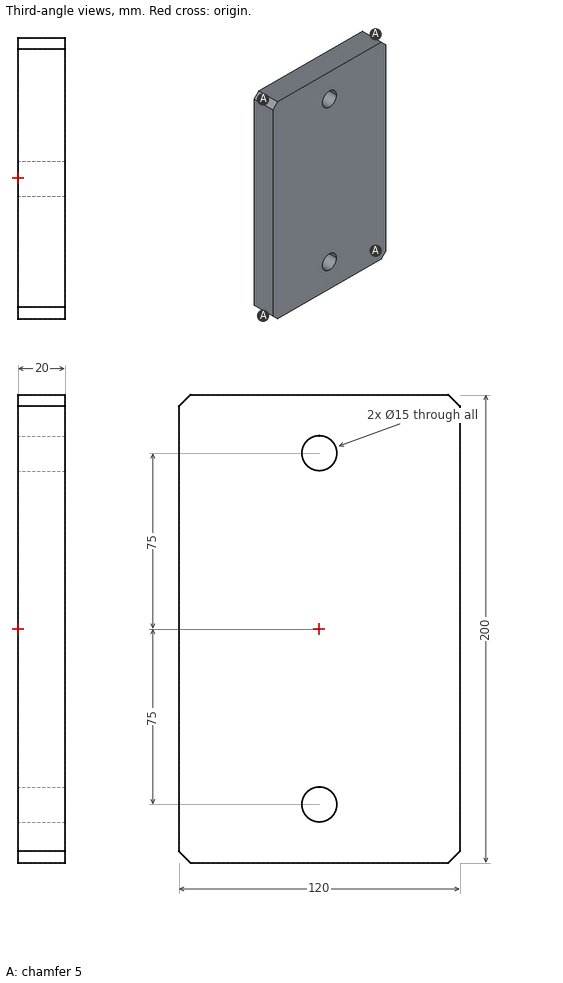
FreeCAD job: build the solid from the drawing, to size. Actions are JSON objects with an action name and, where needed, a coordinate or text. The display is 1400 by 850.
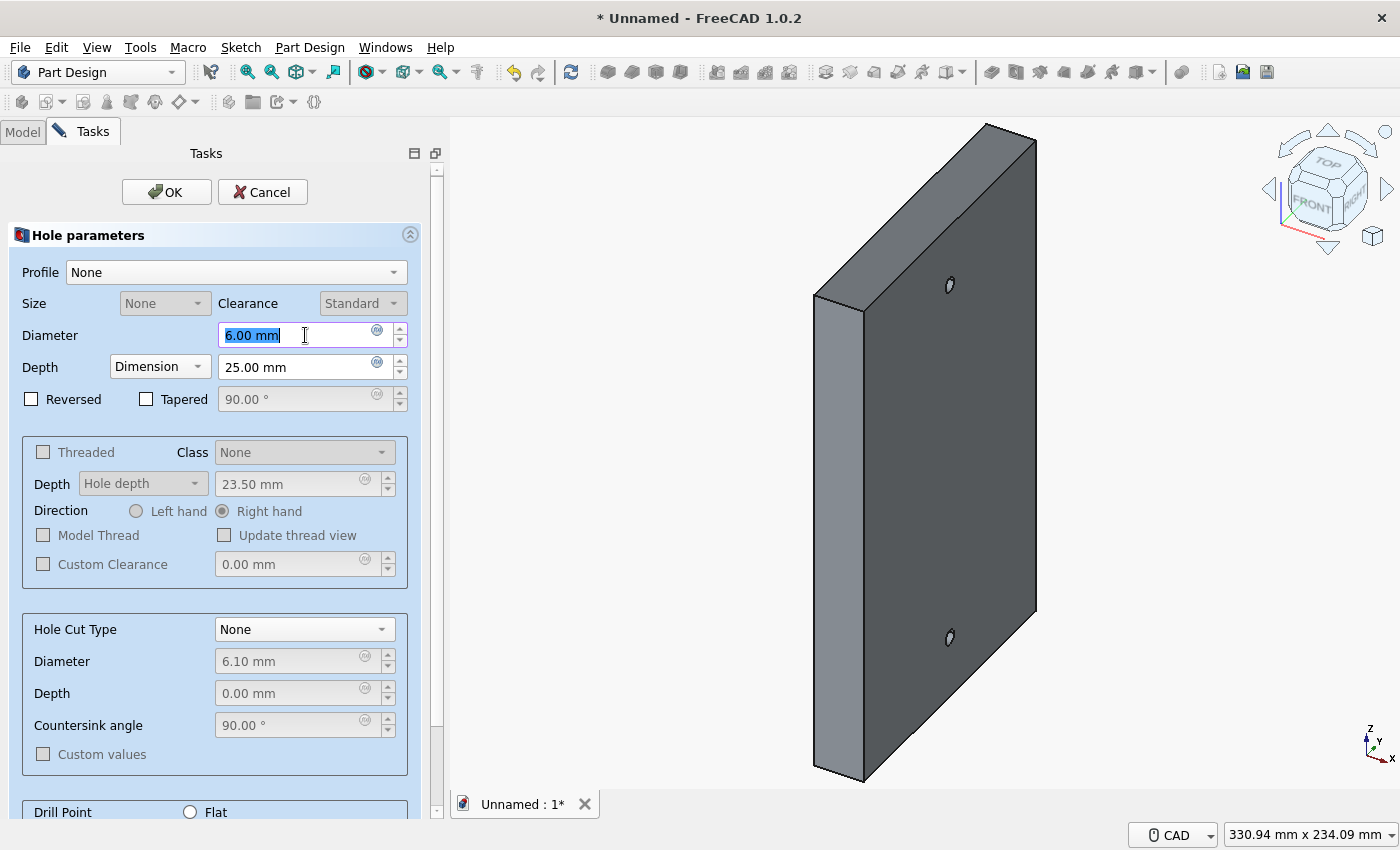
{"action": "type", "text": "15"}
{"action": "key", "text": "Tab"}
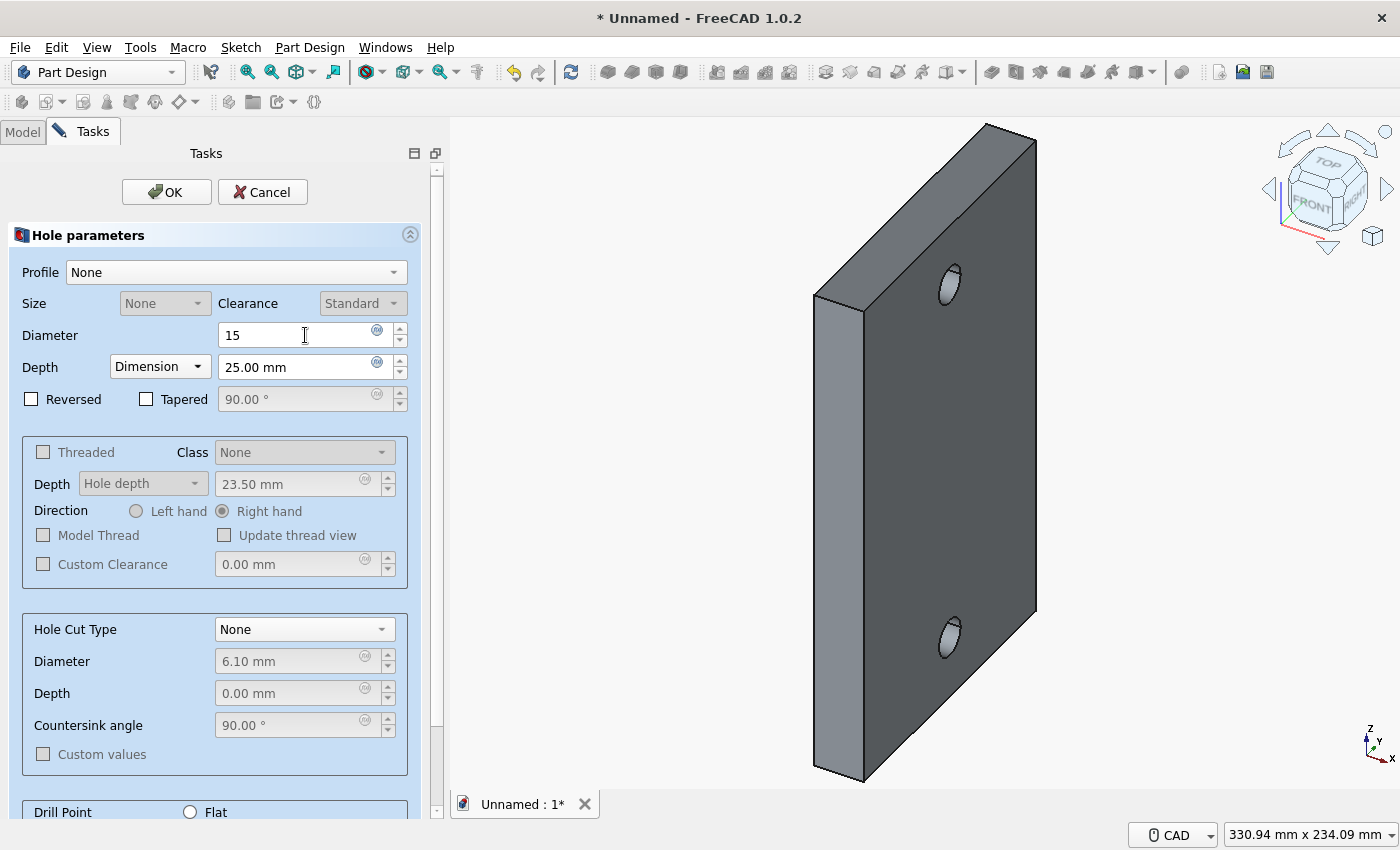
{"action": "left_click", "coordinate": [161, 366]}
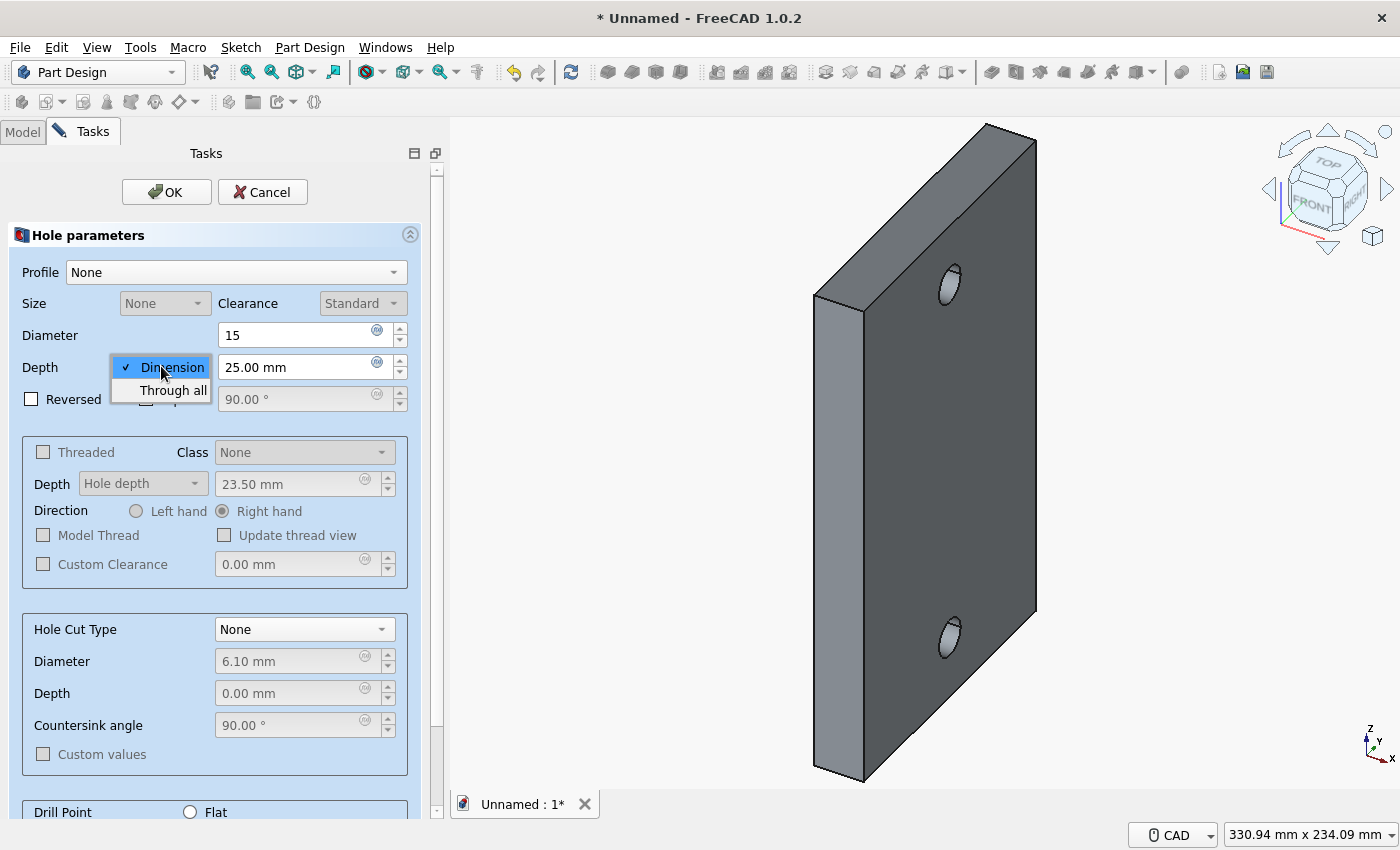
{"action": "left_click", "coordinate": [160, 390]}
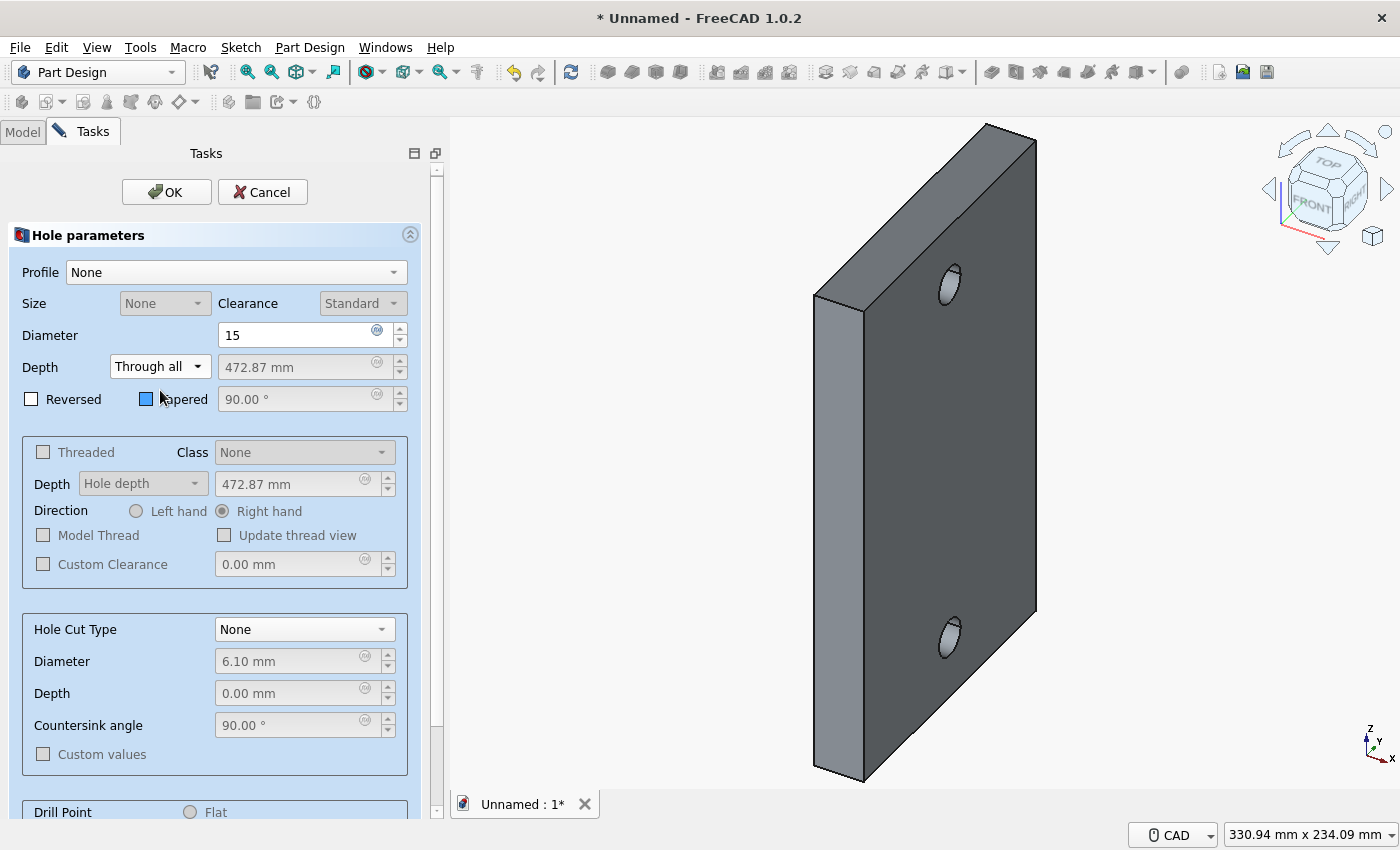
{"action": "left_click", "coordinate": [167, 192]}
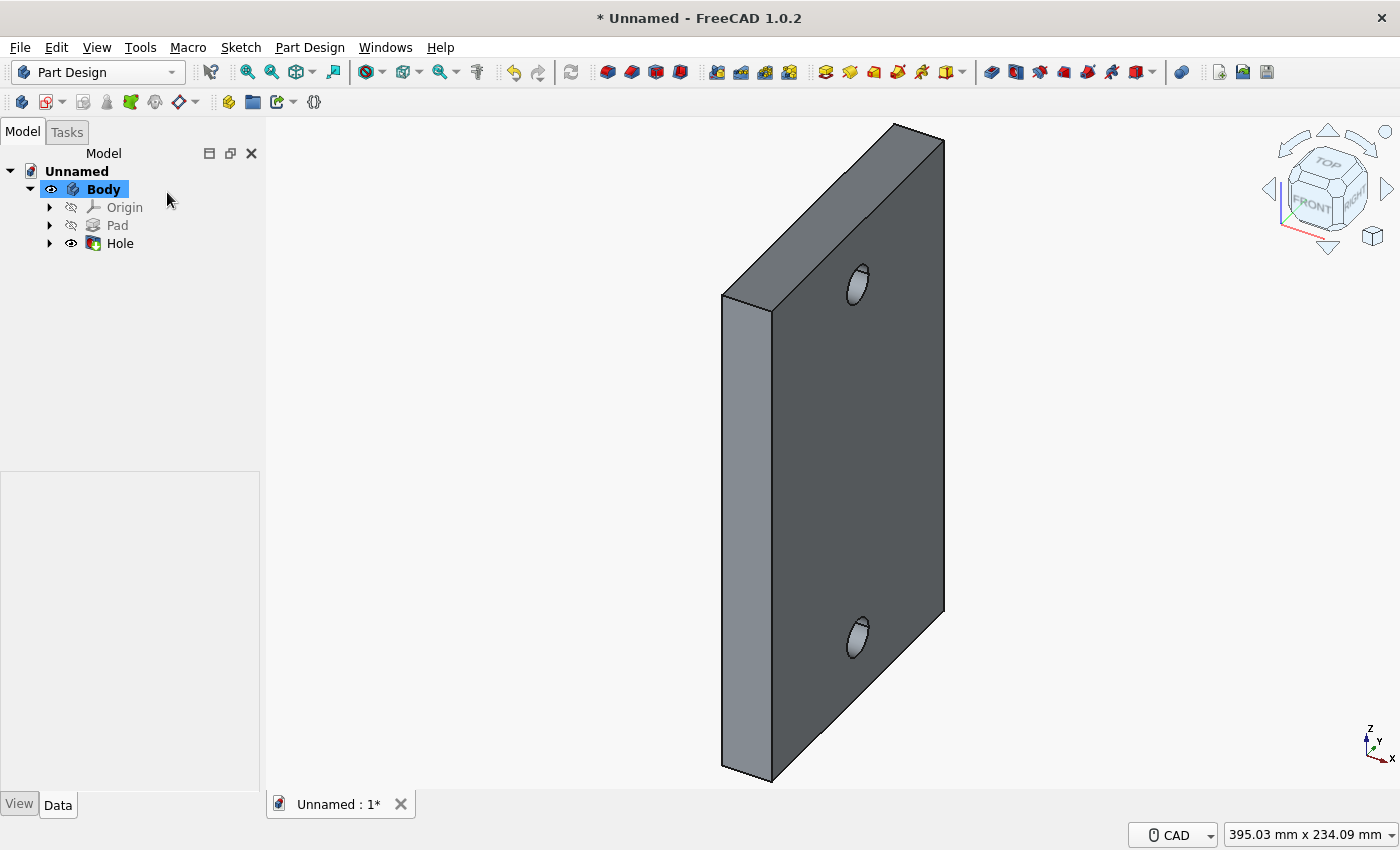
{"action": "left_click", "coordinate": [747, 302]}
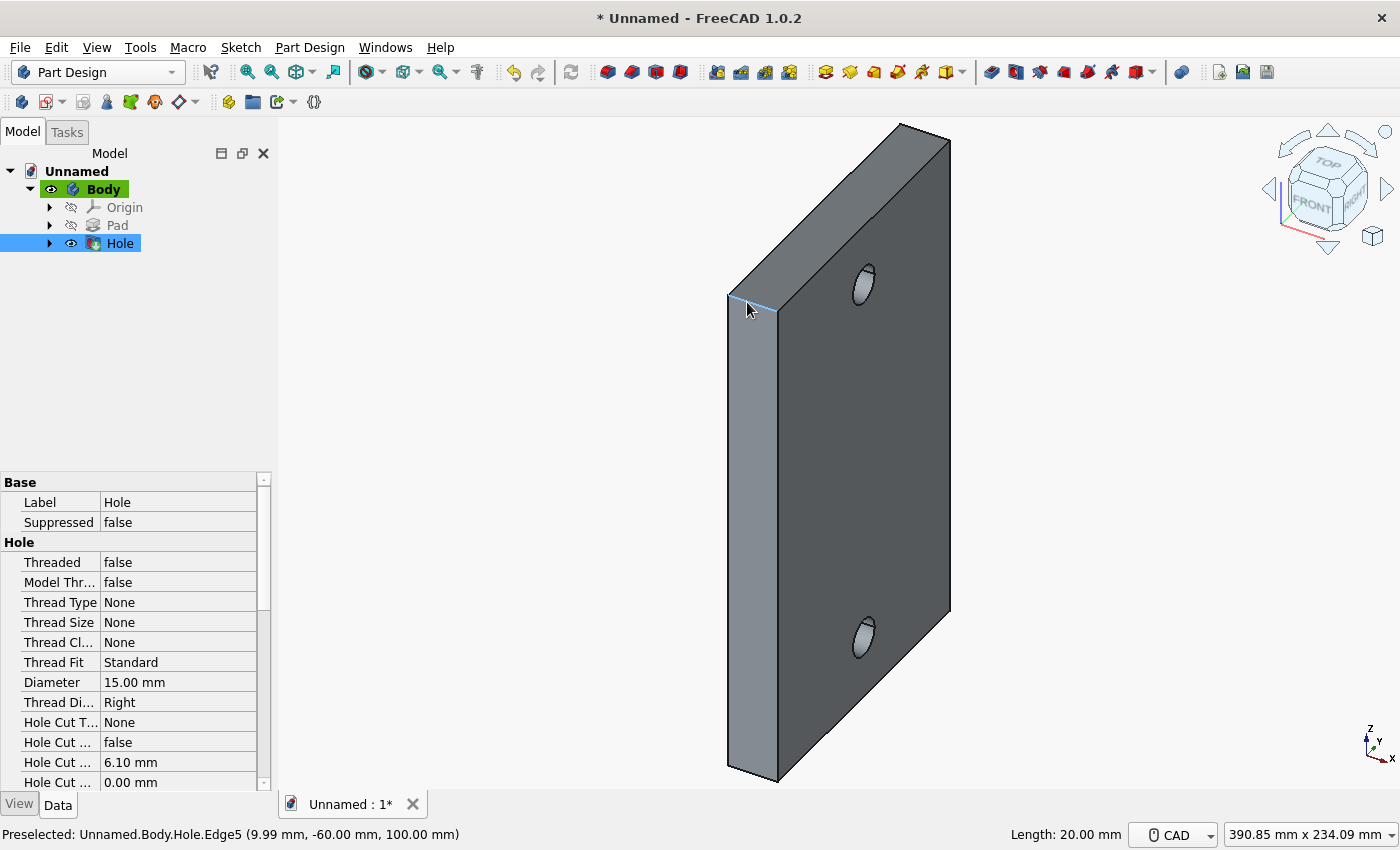
{"action": "key", "text": "0"}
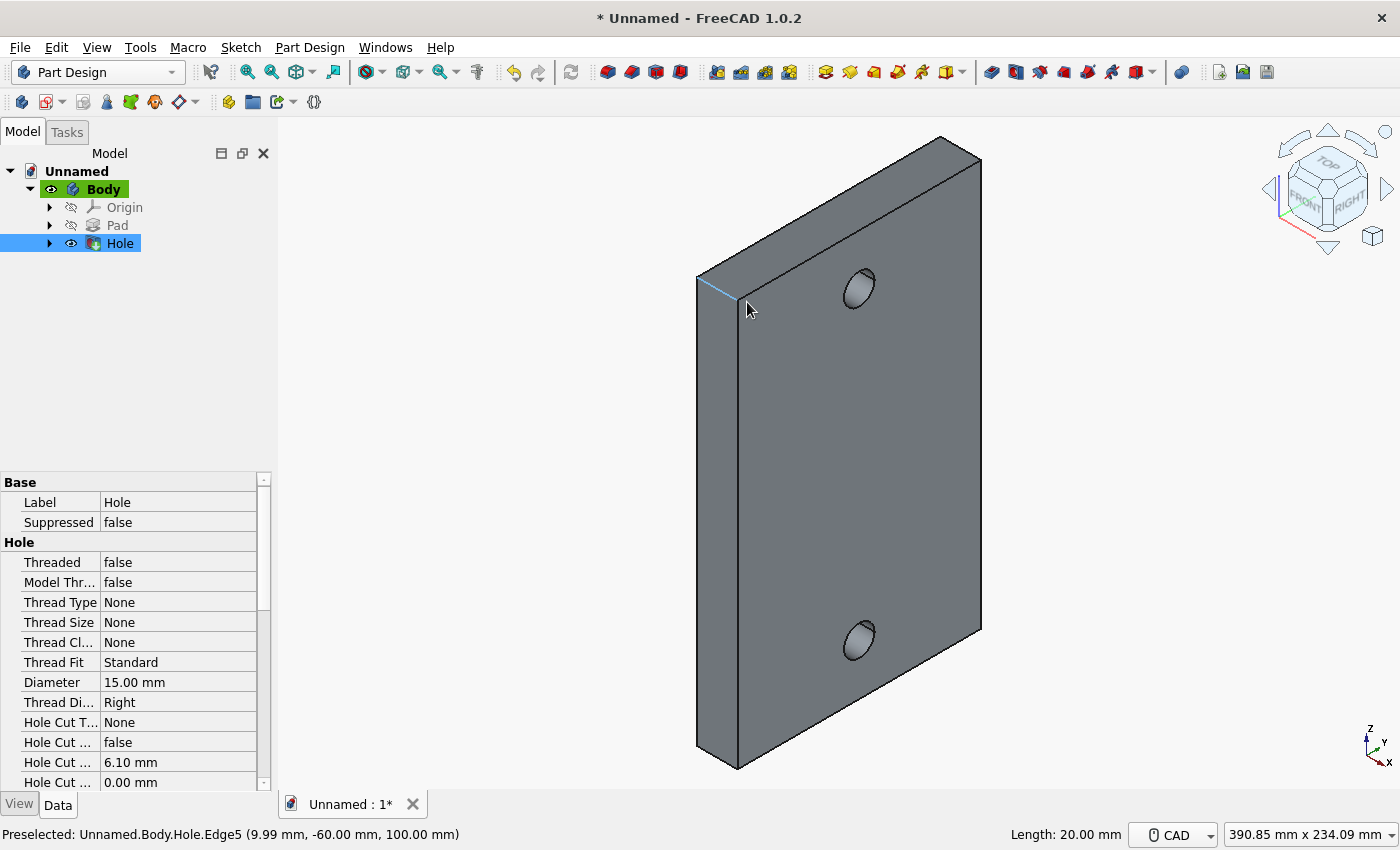
{"action": "key", "text": "2"}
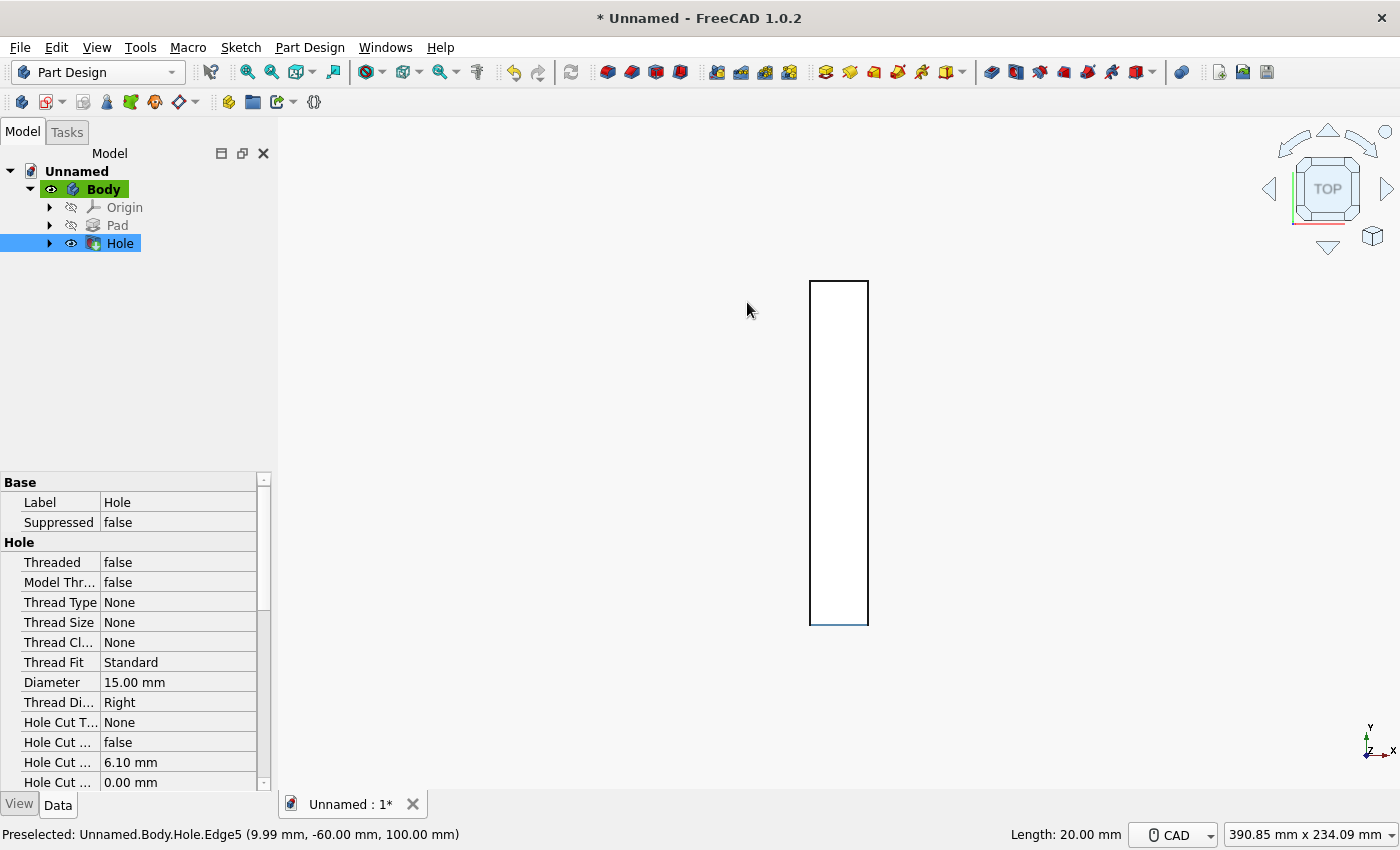
{"action": "left_click", "coordinate": [839, 280], "text": "ctrl"}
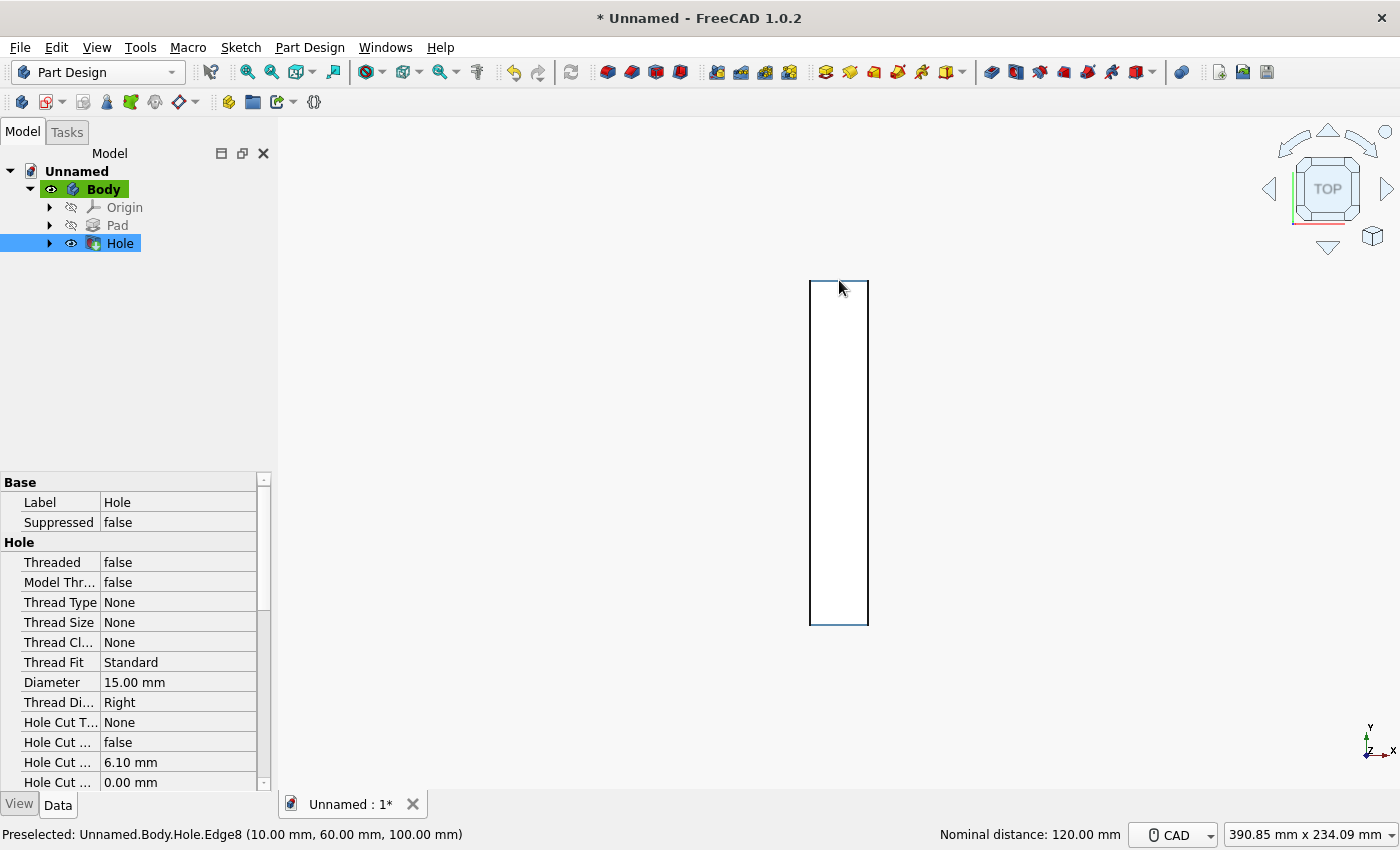
{"action": "key", "text": "1"}